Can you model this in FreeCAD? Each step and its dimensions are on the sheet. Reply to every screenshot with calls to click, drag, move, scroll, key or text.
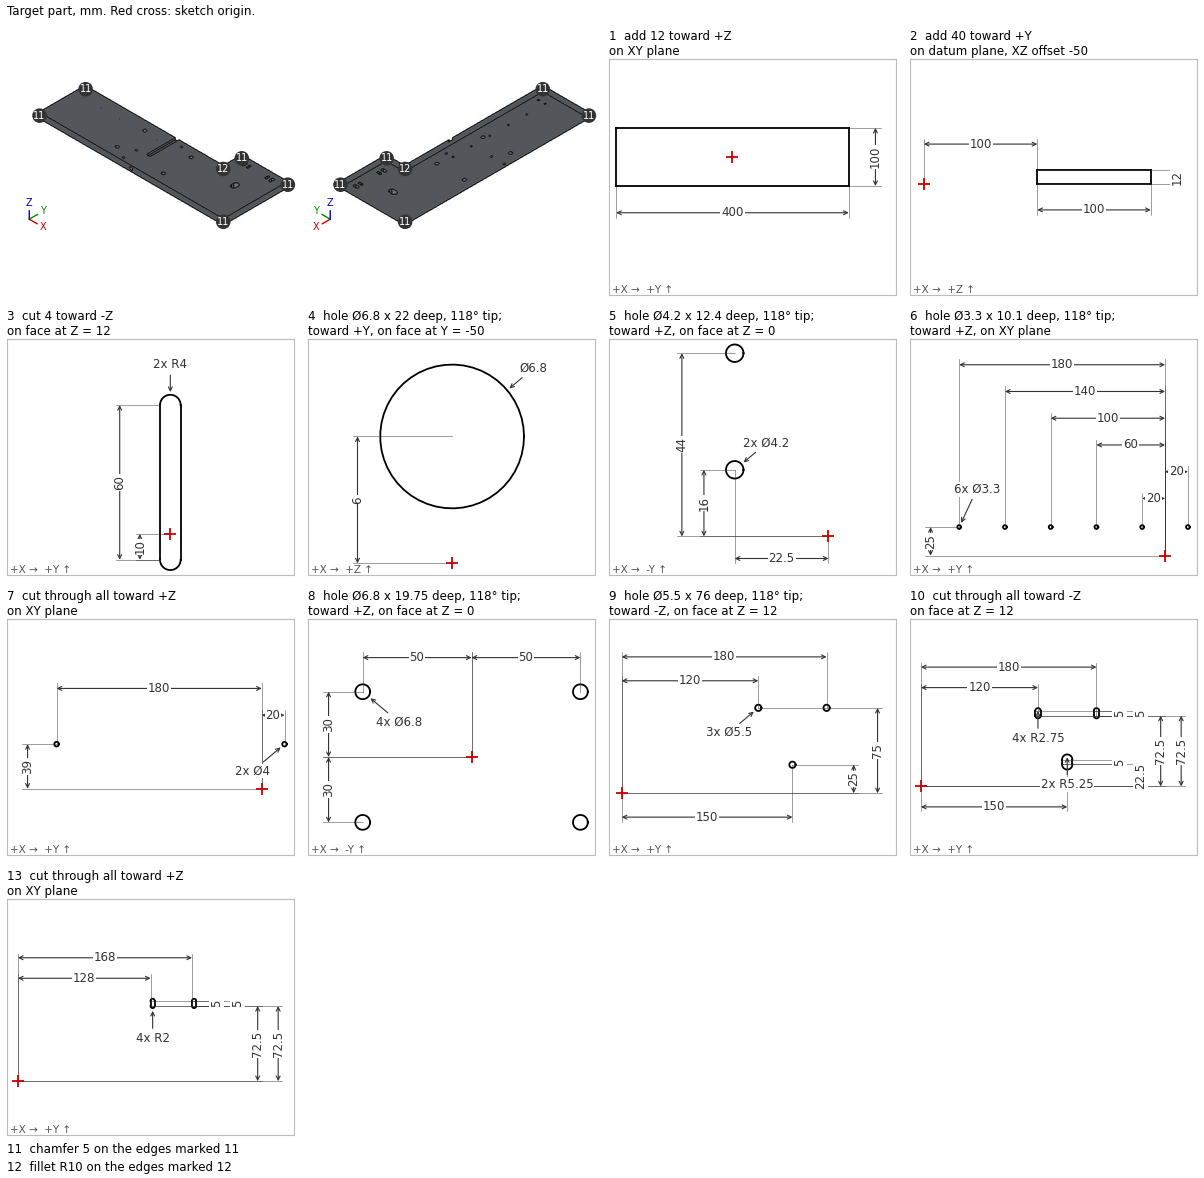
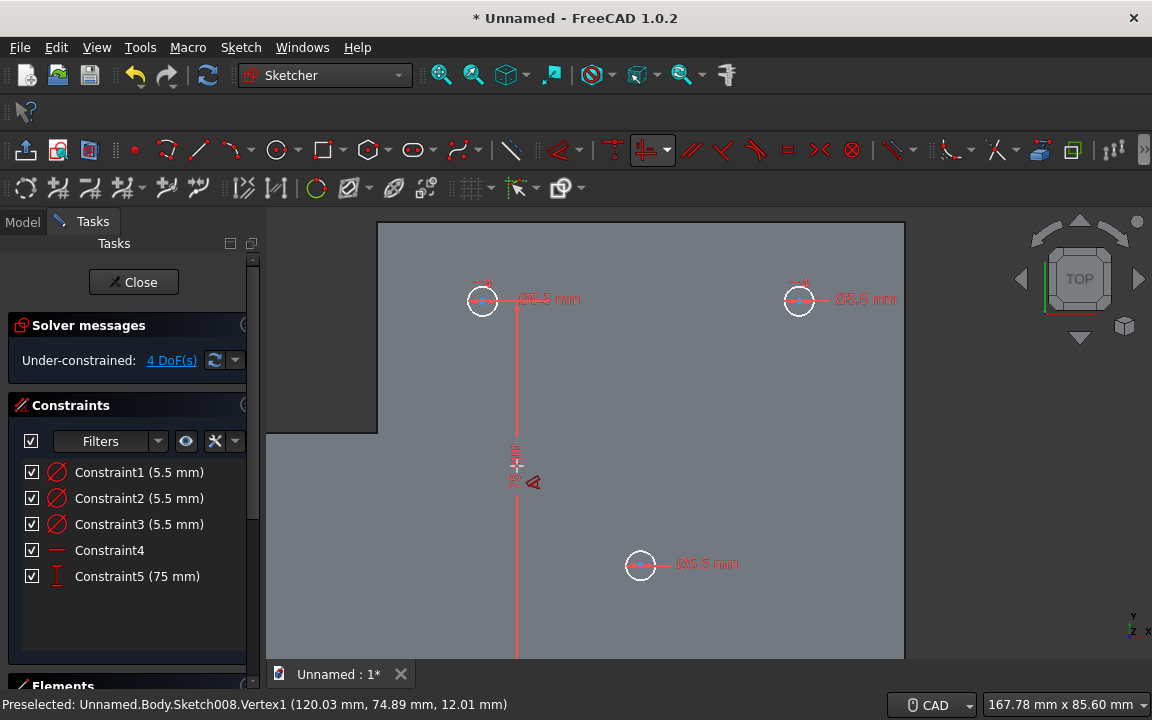
click(641, 566)
click(675, 598)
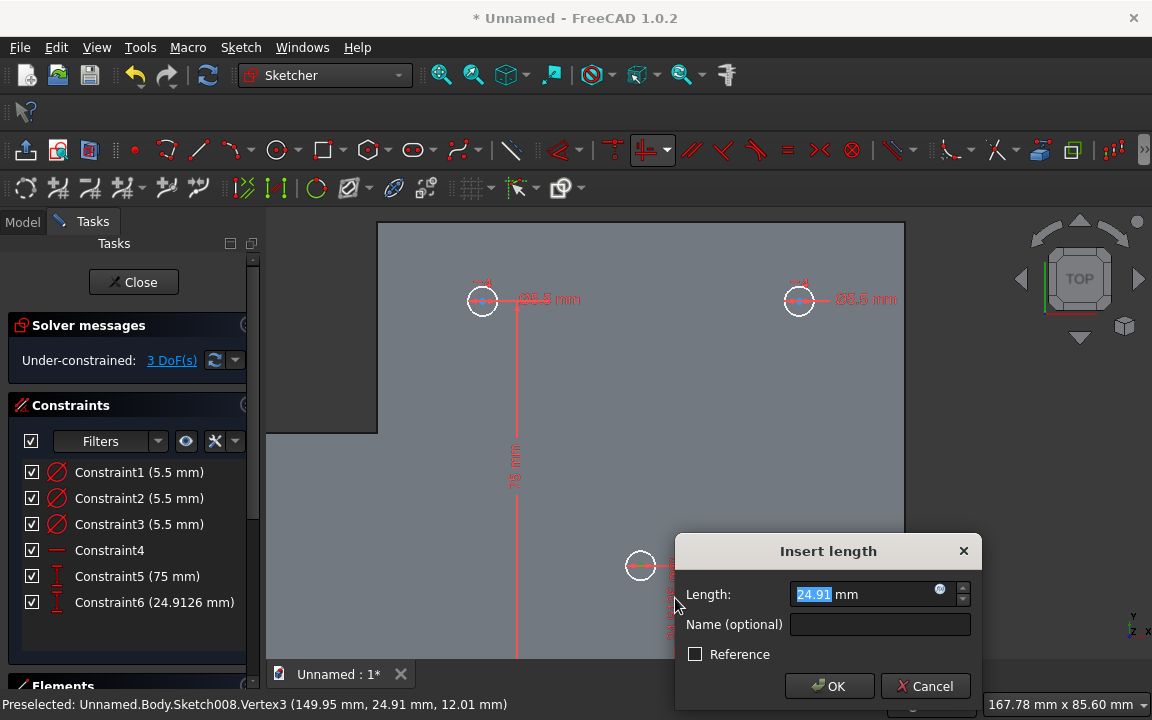
text(25)
key(Return)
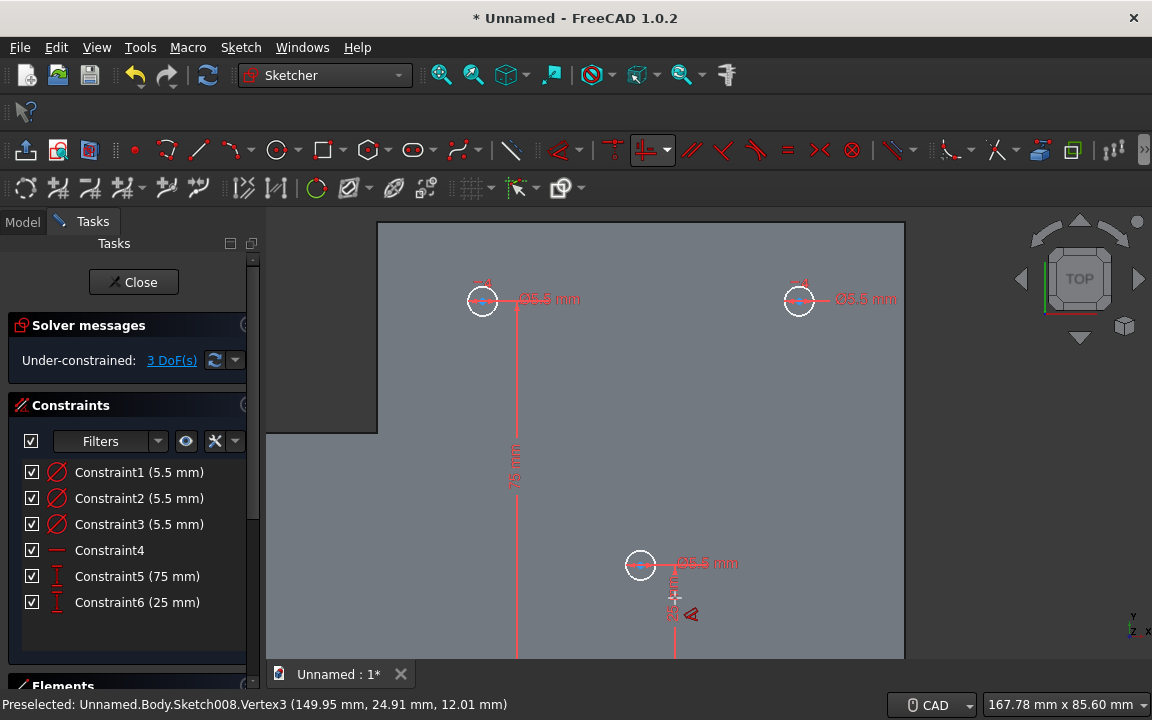
click(483, 301)
click(388, 267)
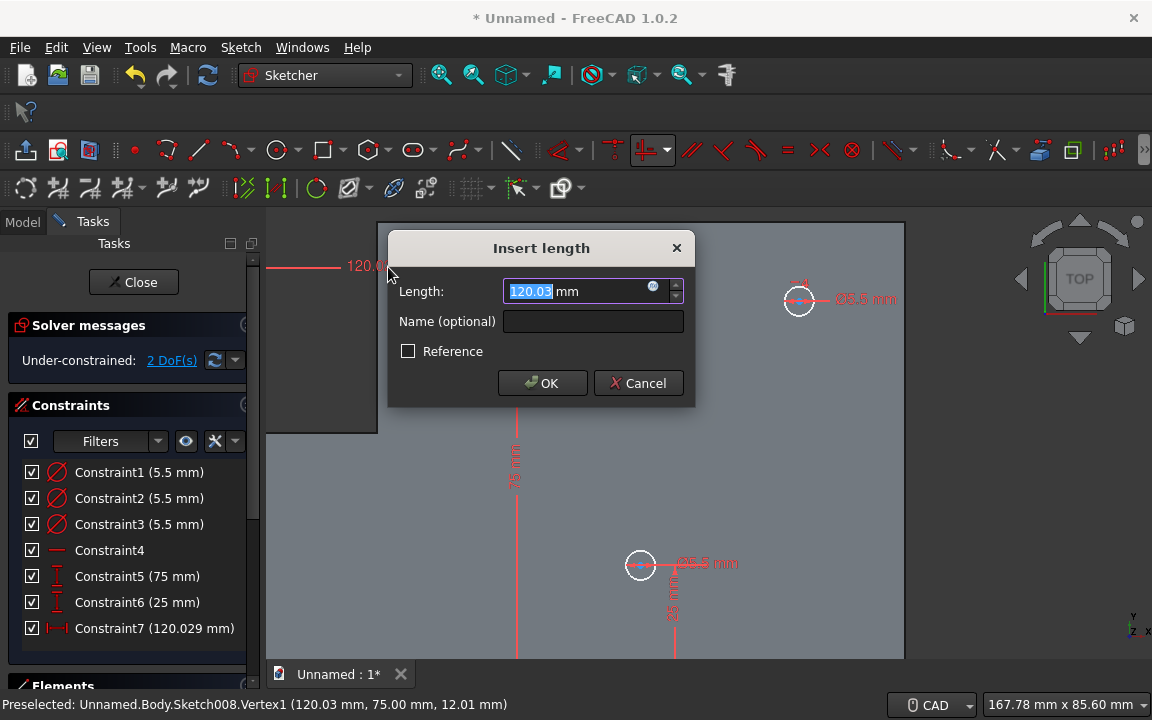
text(120)
key(Return)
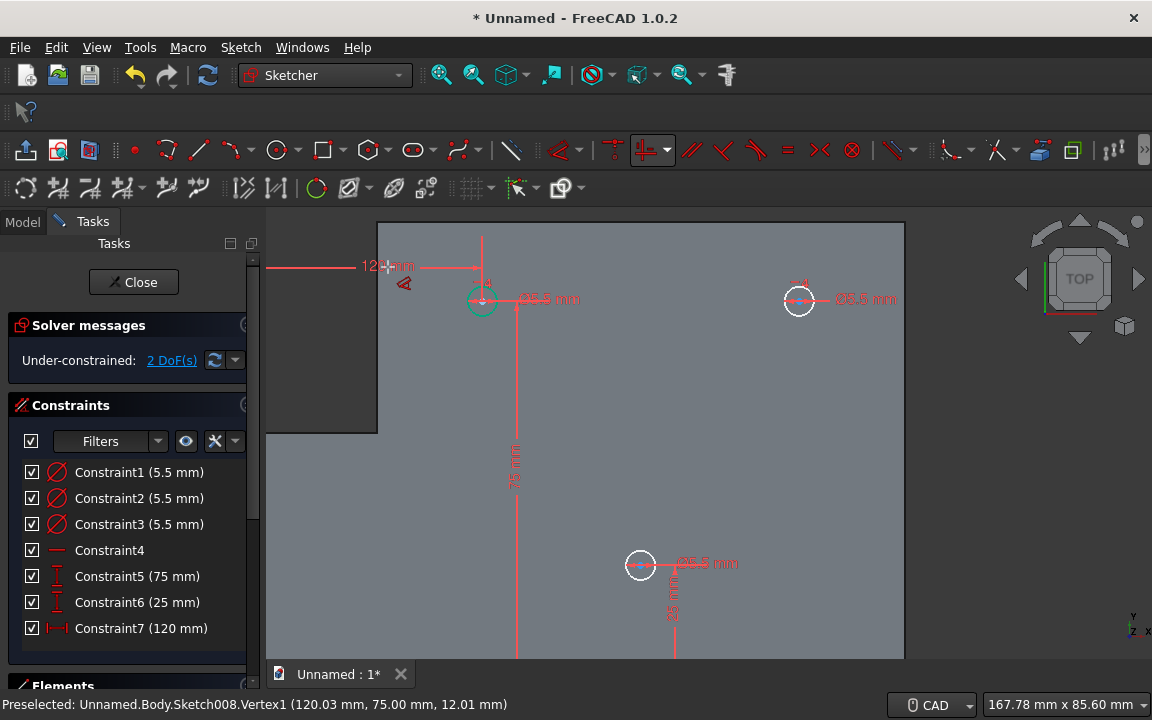
click(799, 301)
click(547, 267)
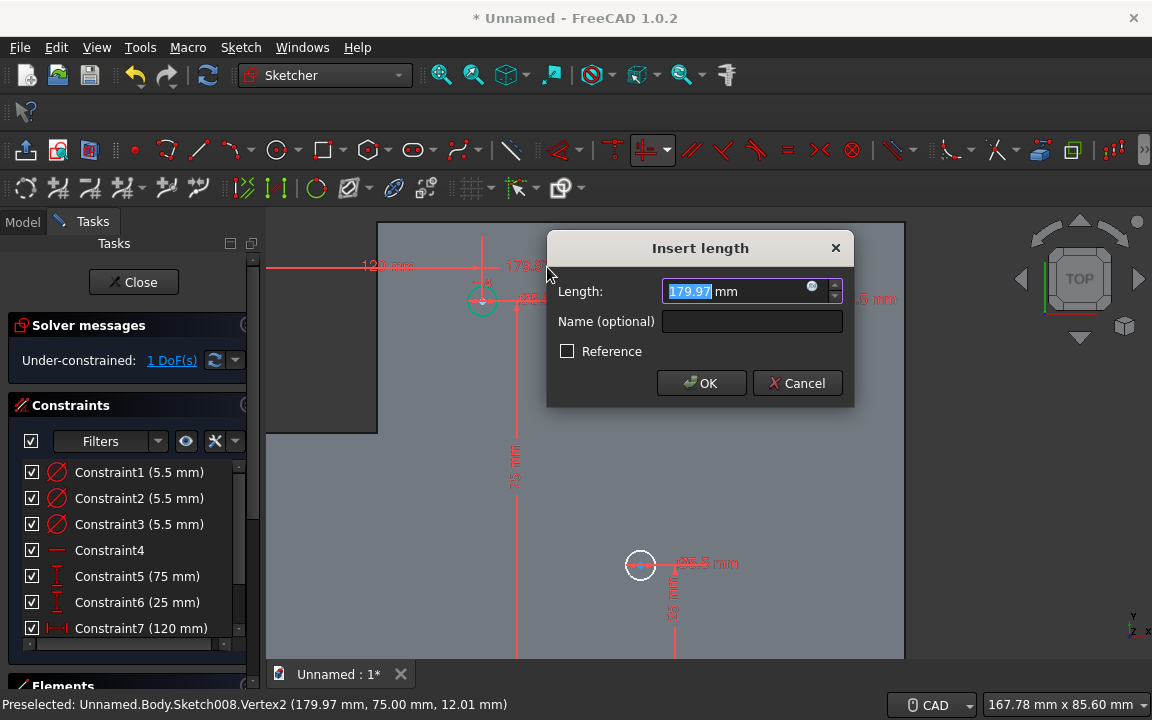
text(180)
key(Return)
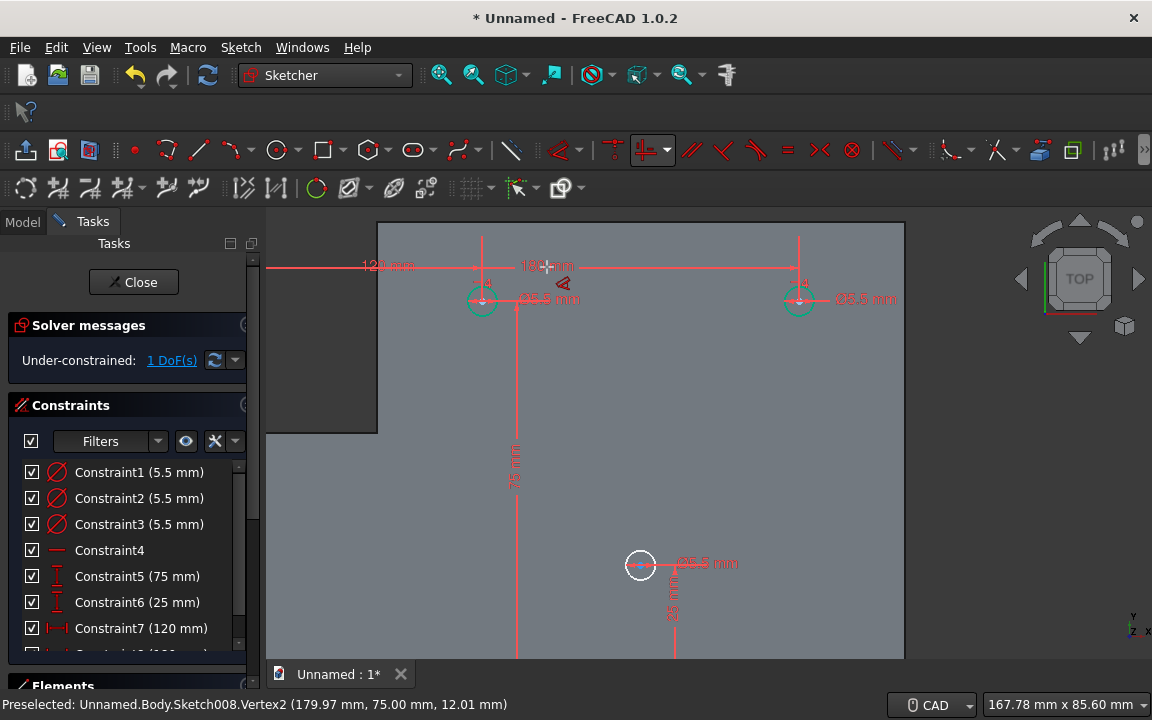
click(641, 565)
click(467, 531)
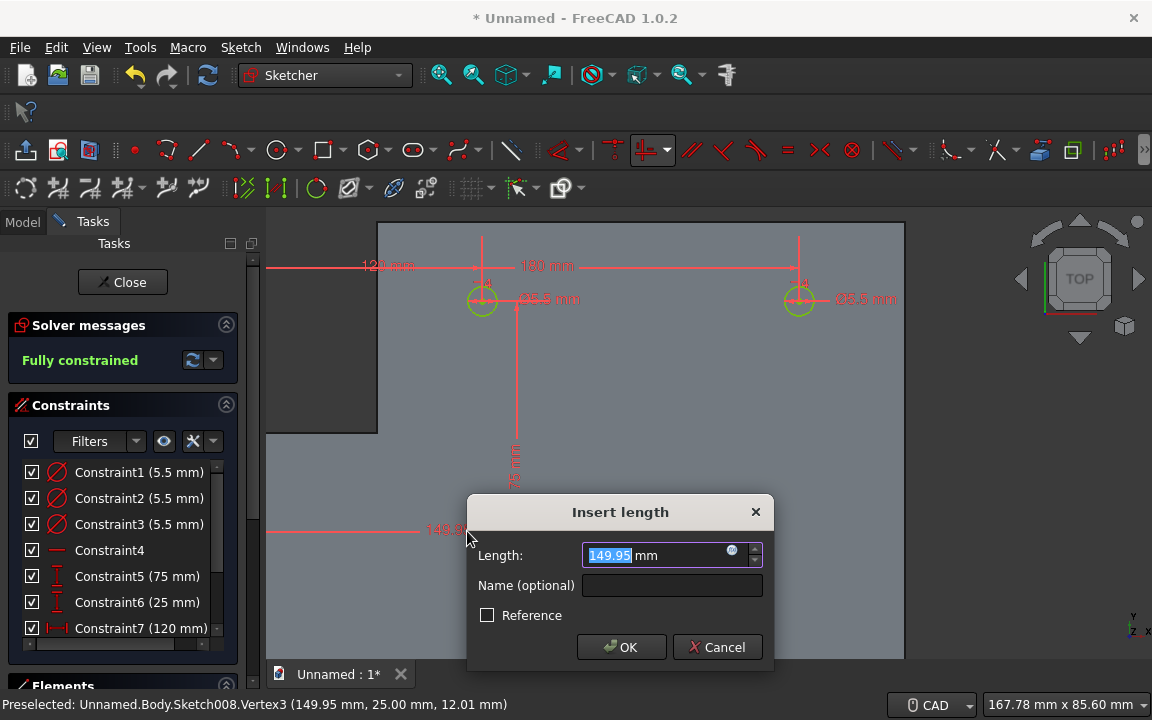
text(150)
key(Return)
key(Escape)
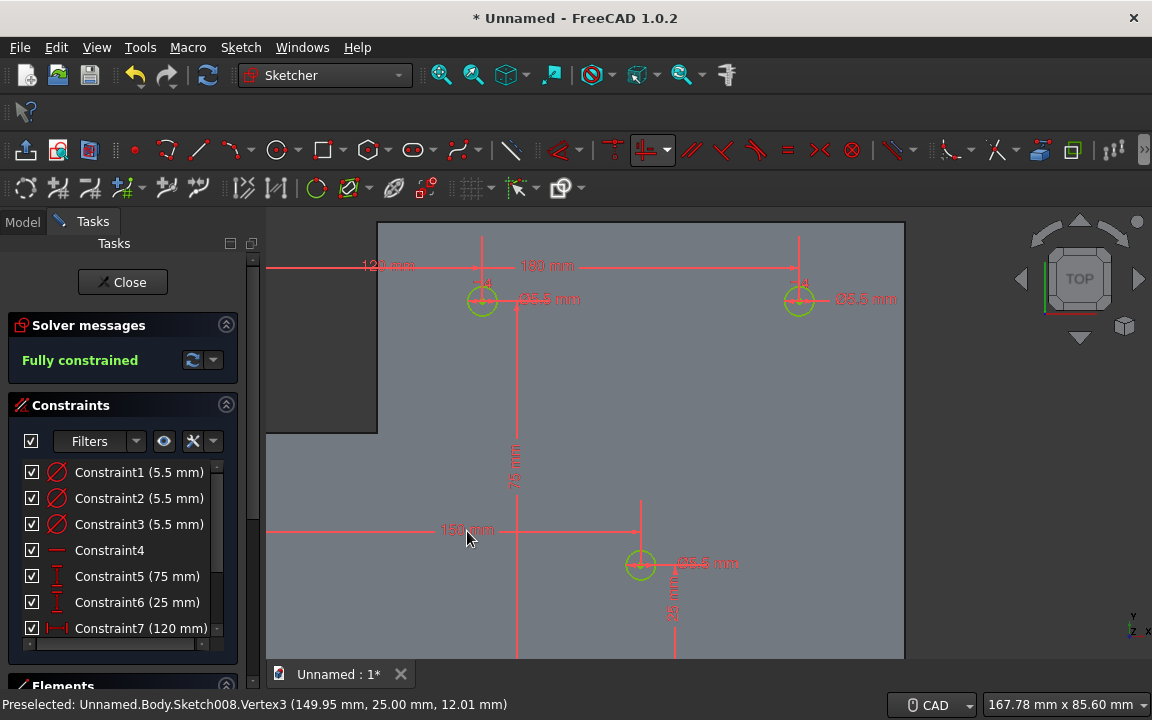
click(123, 282)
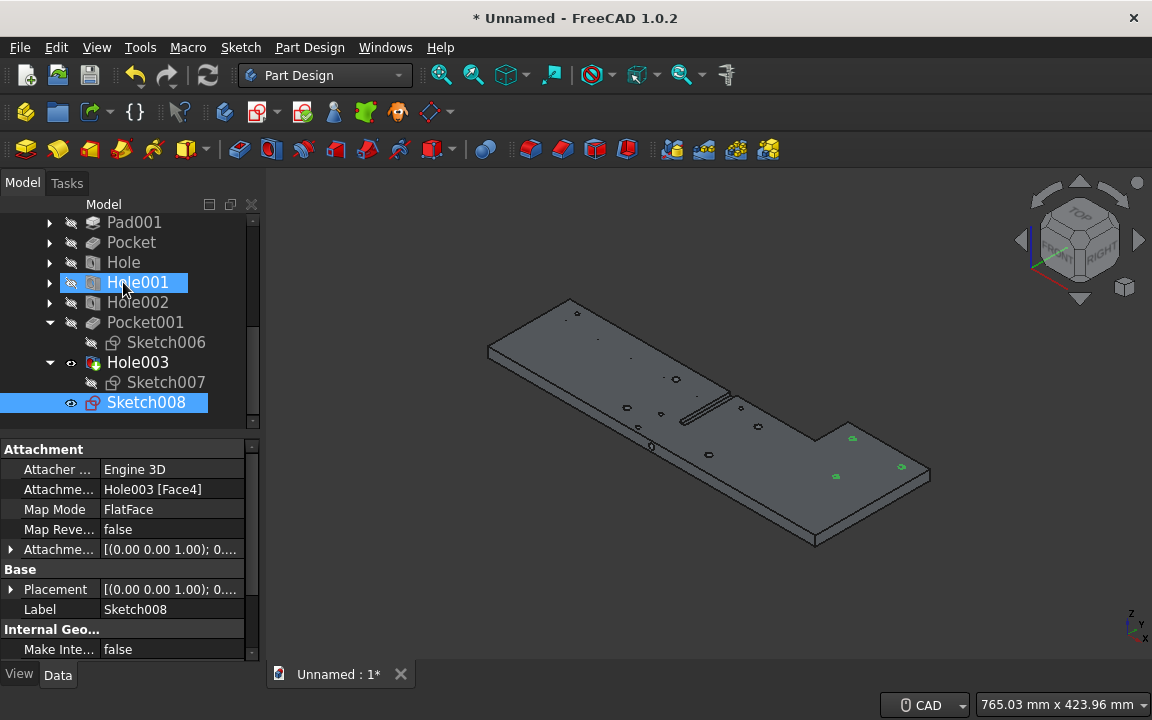
click(272, 150)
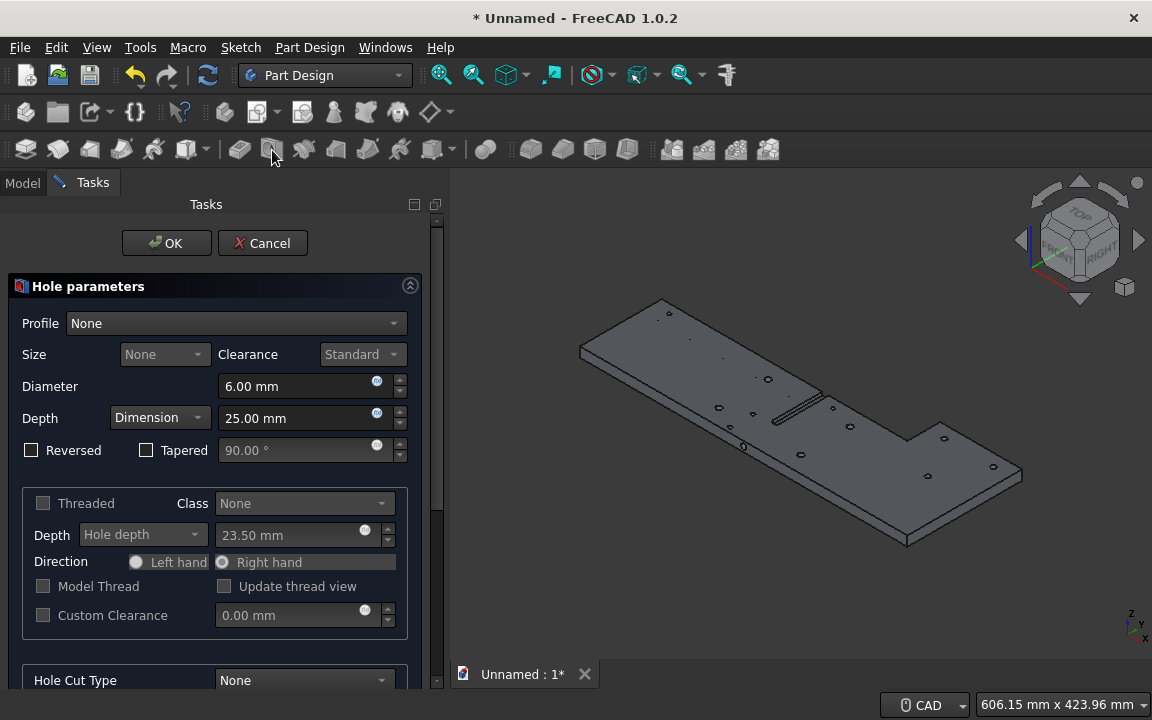
triple_click(305, 386)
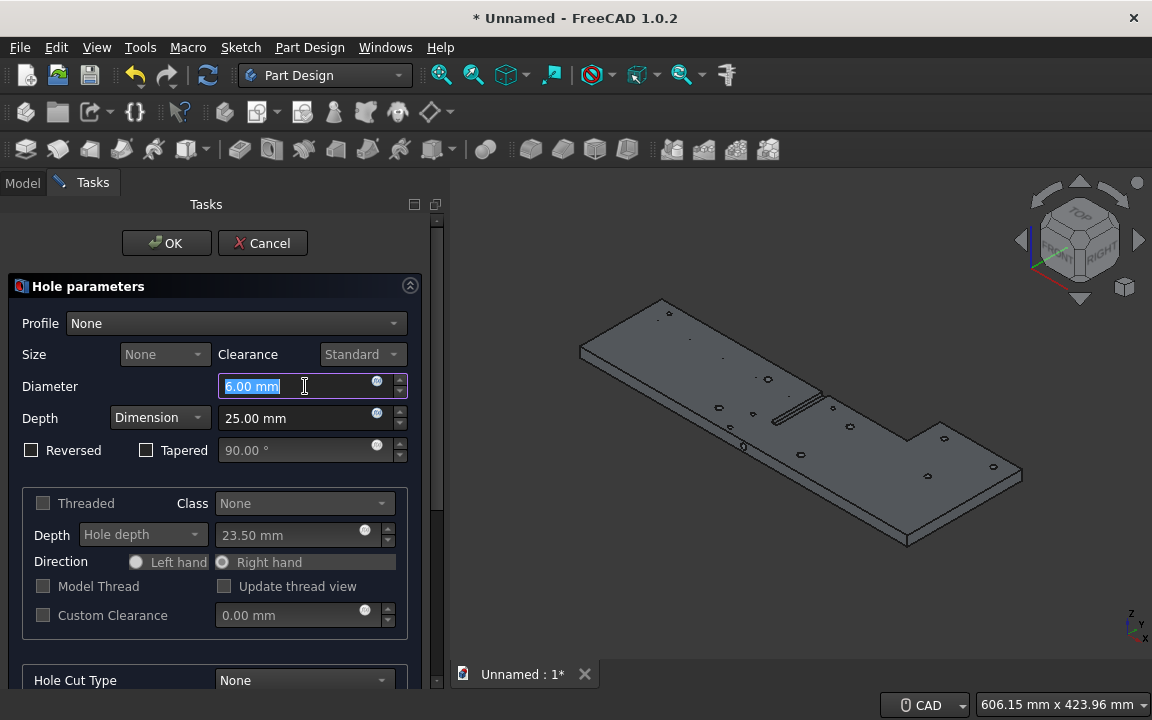
text(5.5)
key(Tab)